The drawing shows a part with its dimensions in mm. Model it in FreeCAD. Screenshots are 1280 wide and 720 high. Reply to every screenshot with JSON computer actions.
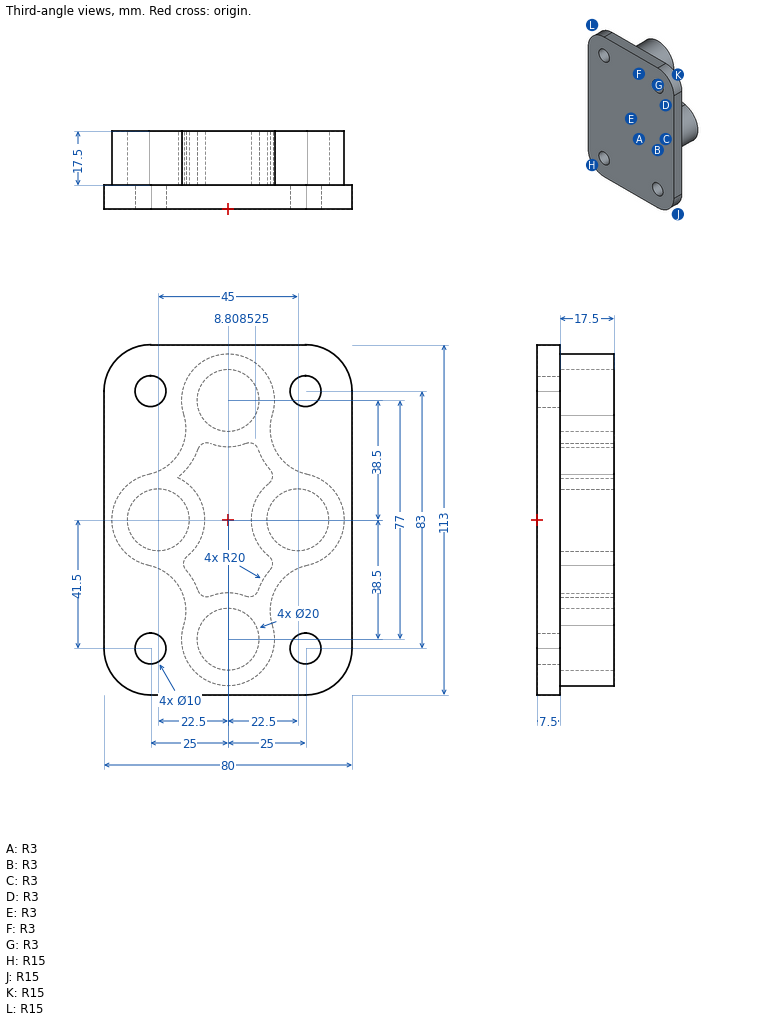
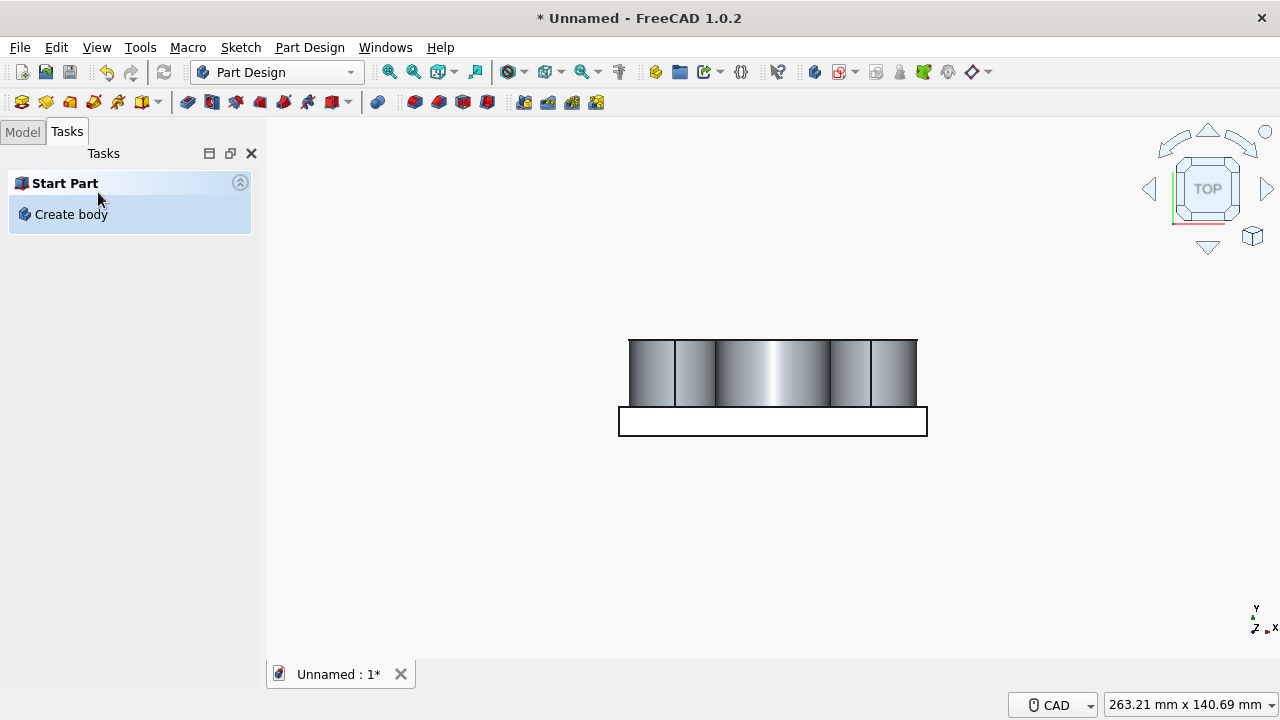
{"action": "left_click", "coordinate": [390, 72]}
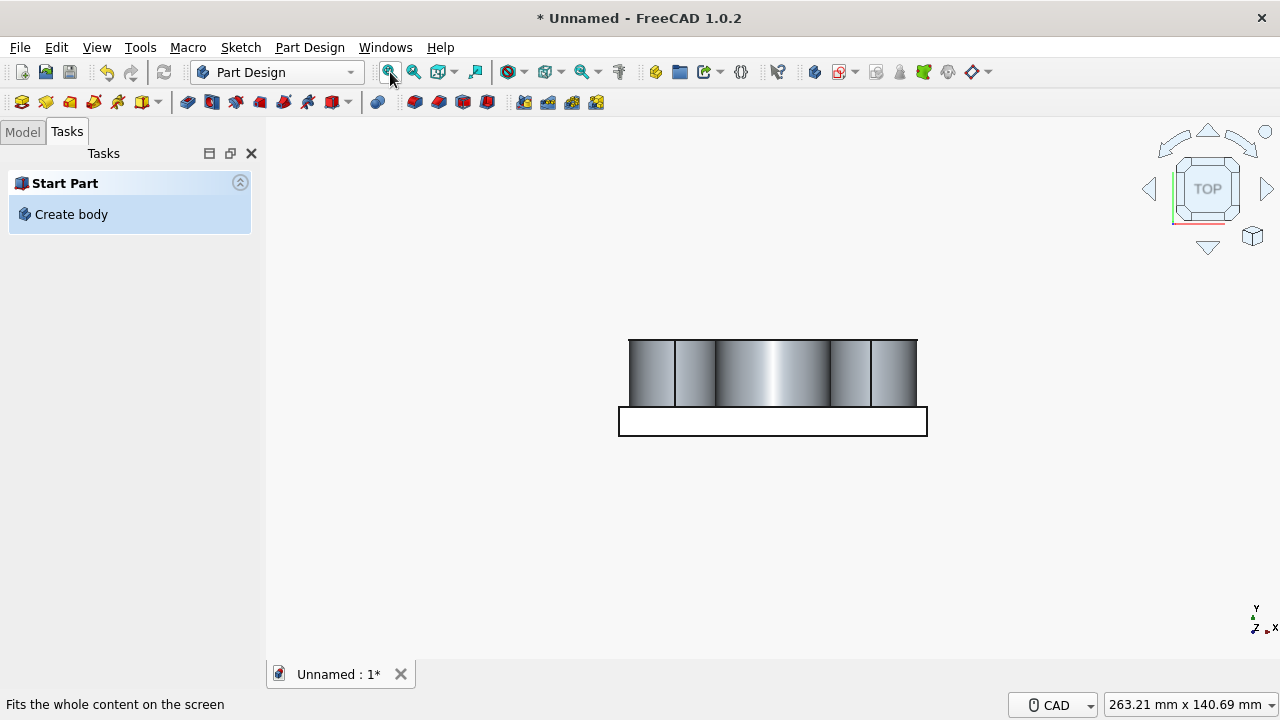
{"action": "key", "text": "0"}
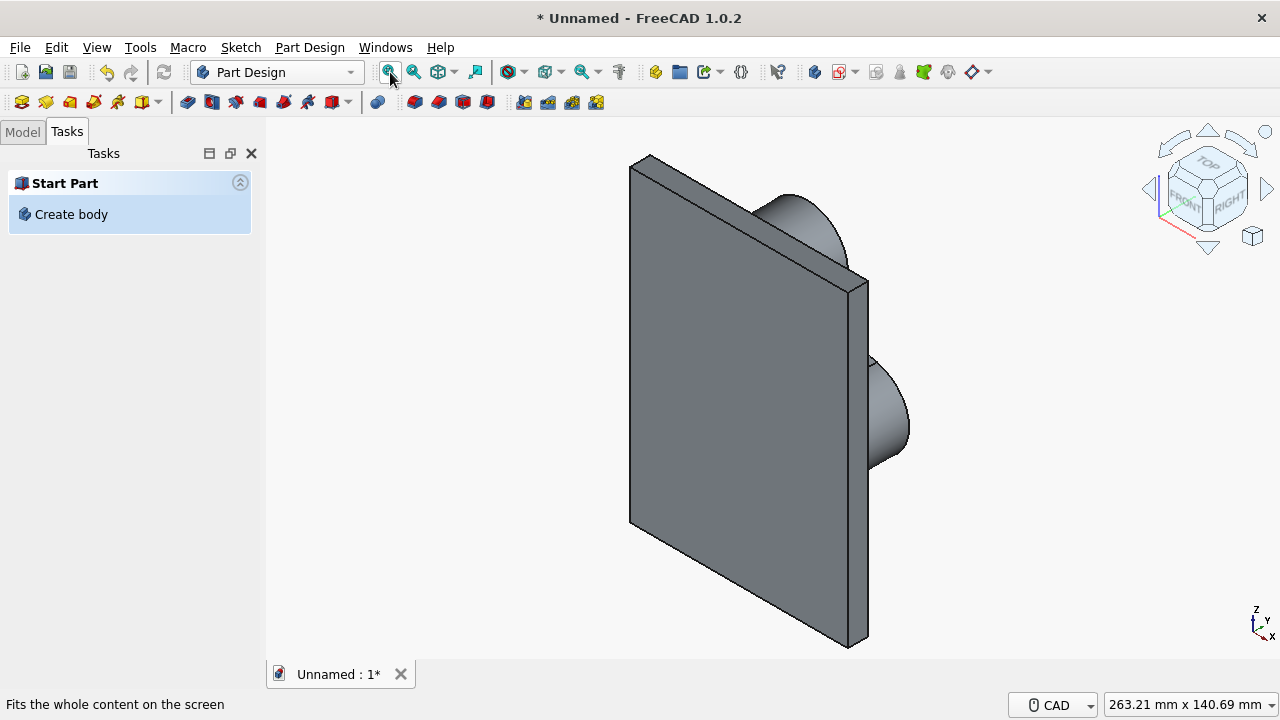
{"action": "key", "text": "1"}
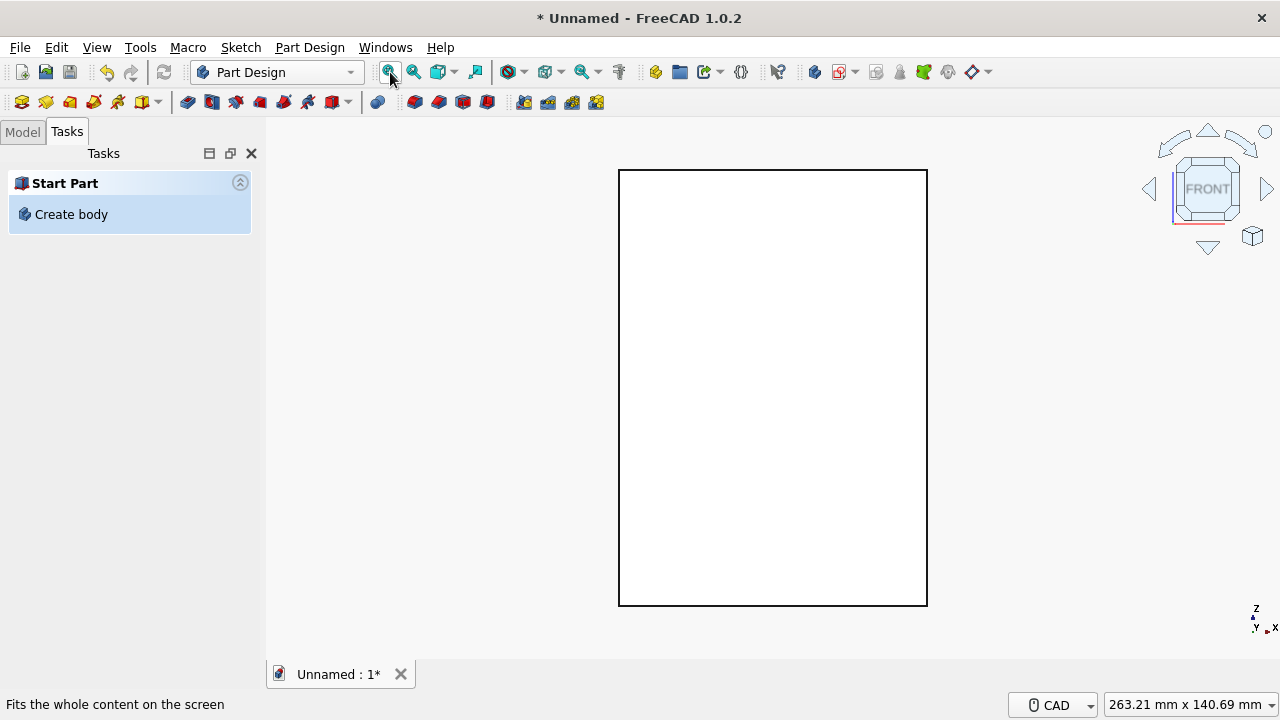
{"action": "key", "text": "3"}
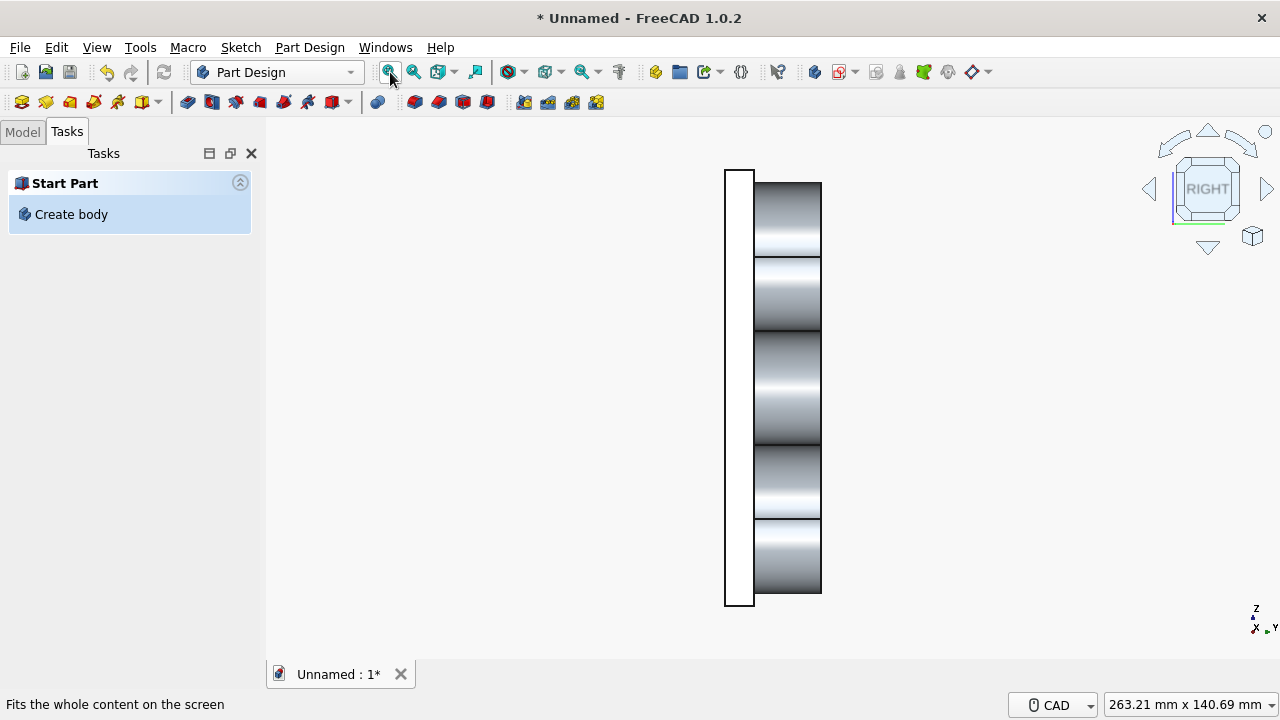
{"action": "key", "text": "5"}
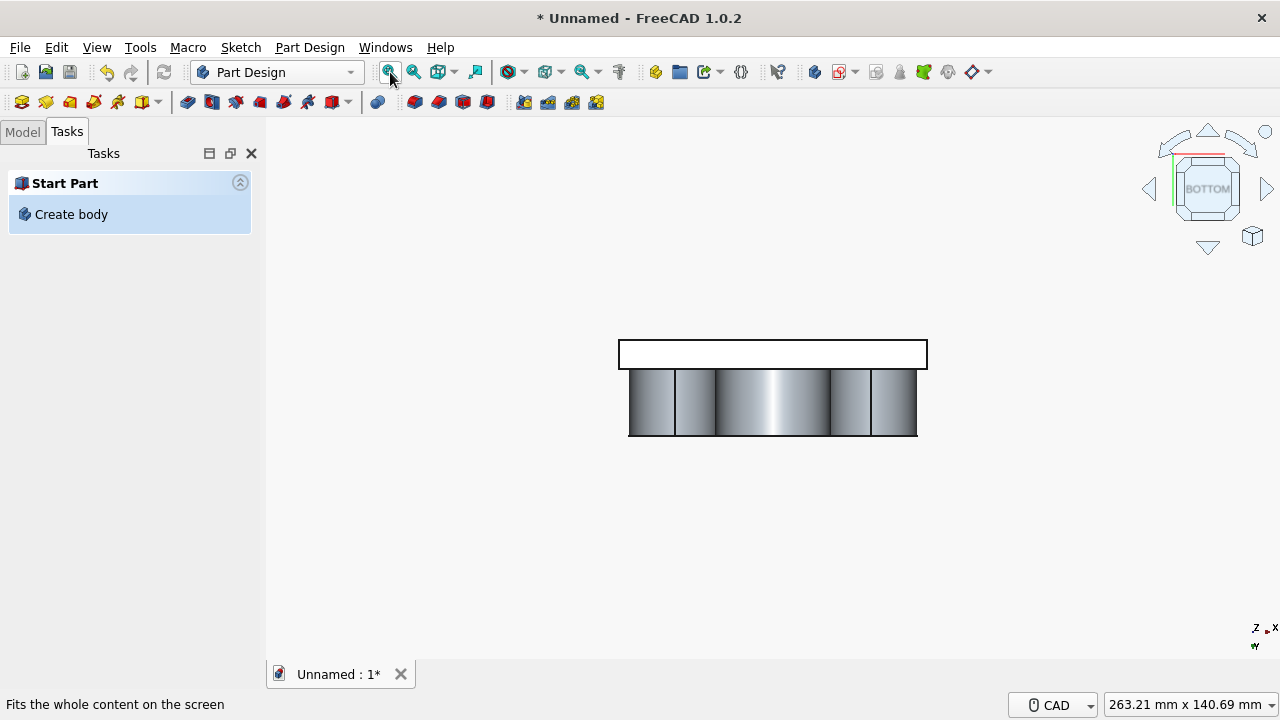
{"action": "left_click", "coordinate": [390, 72]}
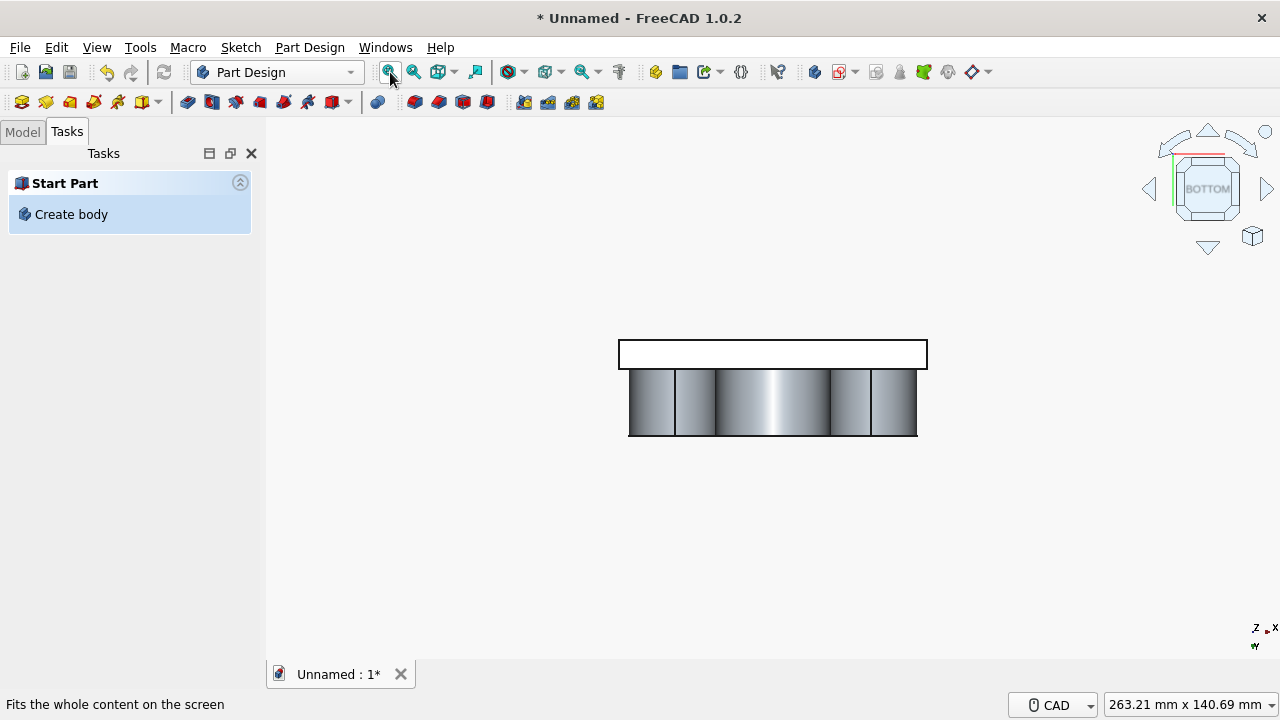
{"action": "key", "text": "4"}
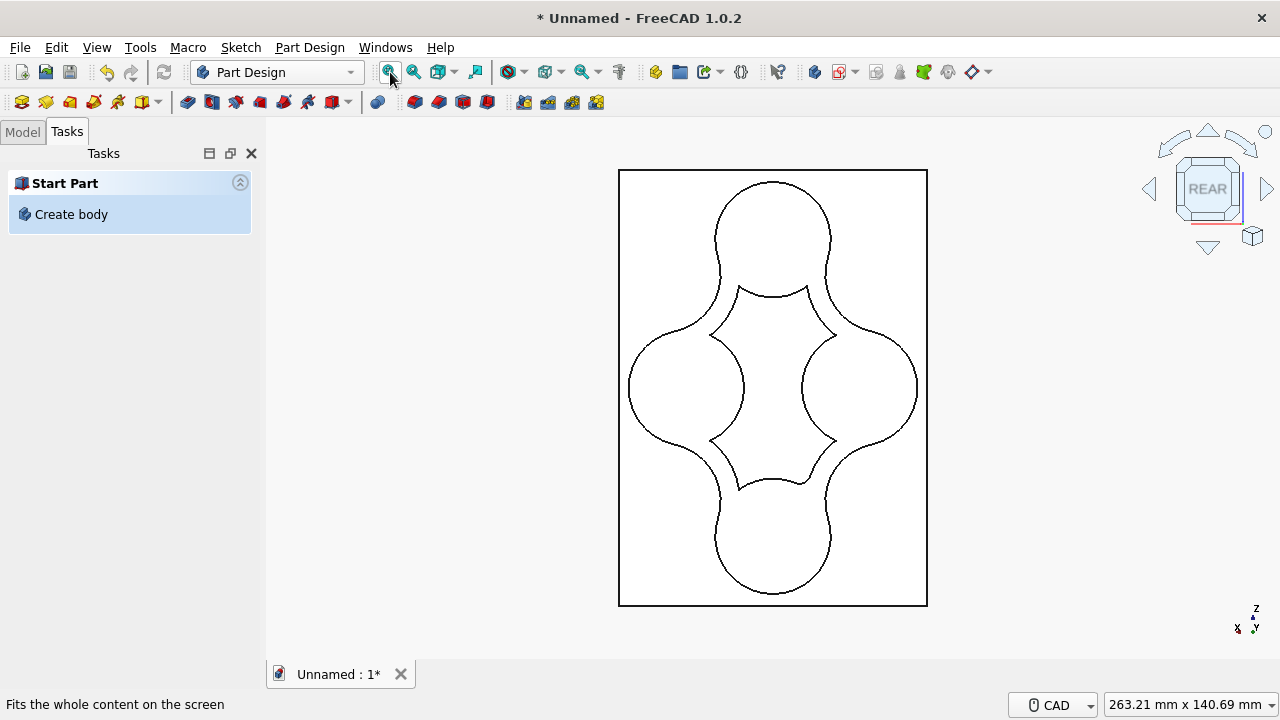
{"action": "key", "text": "6"}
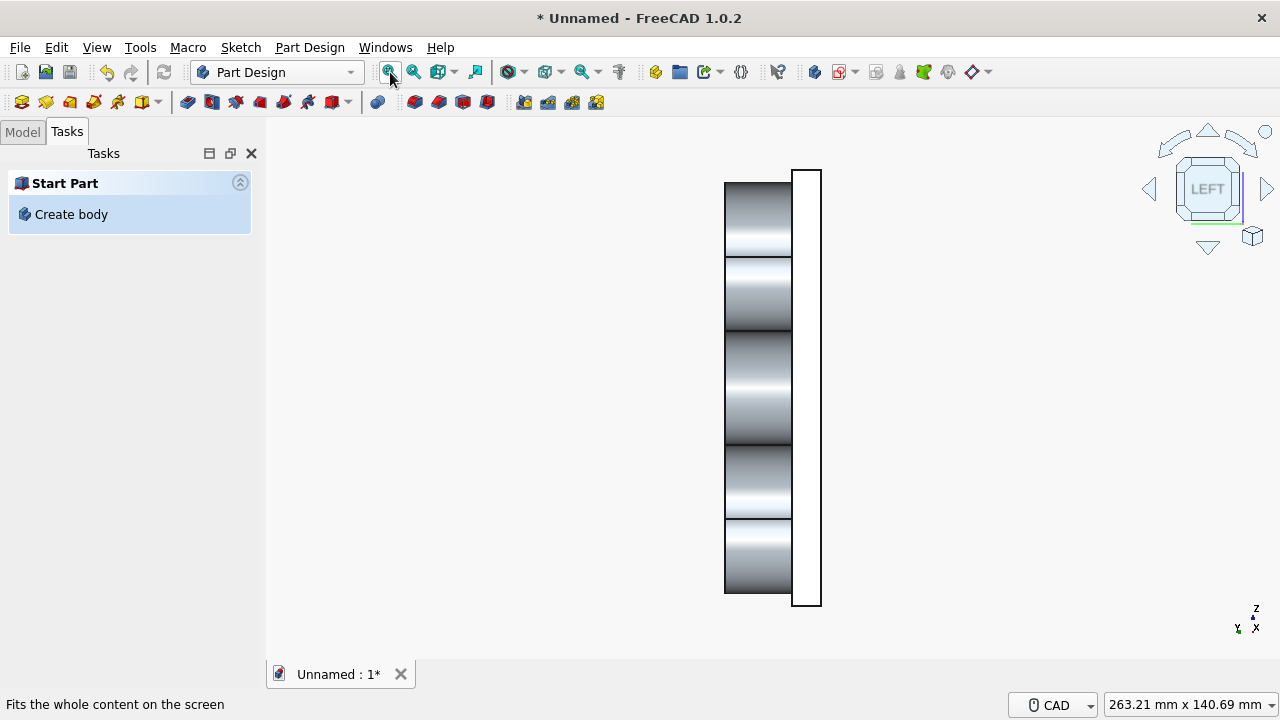
{"action": "key", "text": "v 3"}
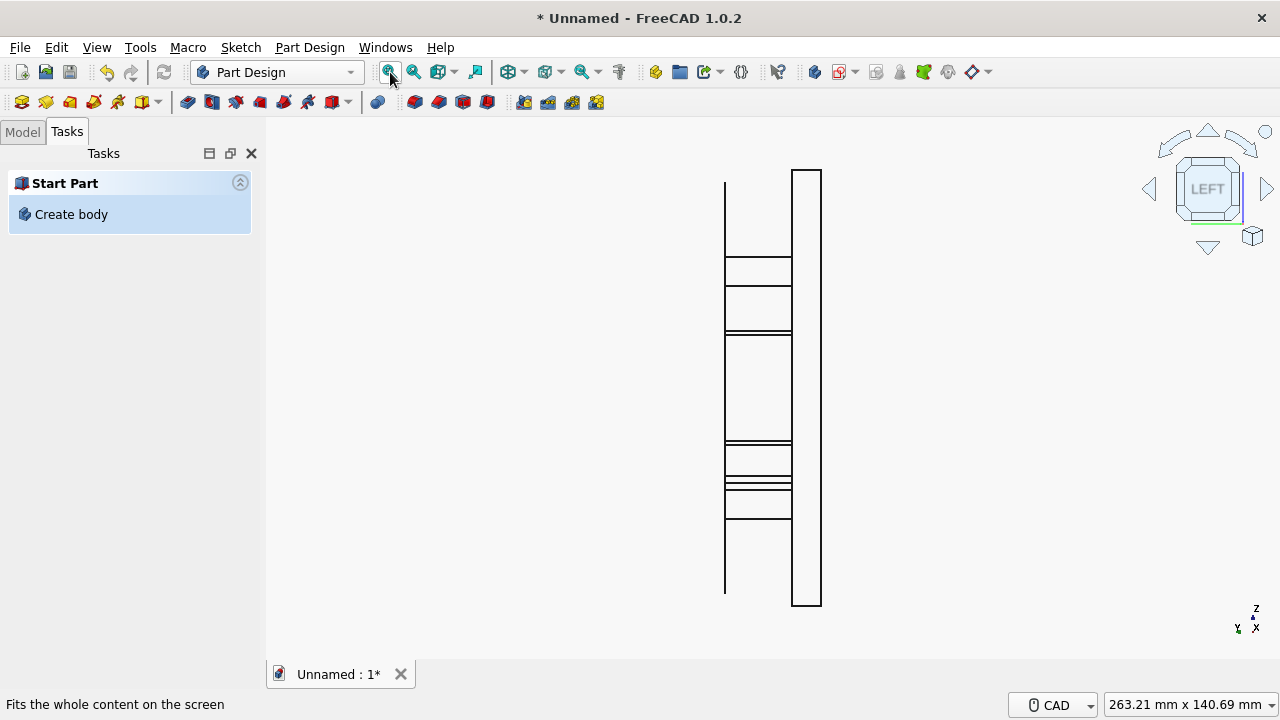
{"action": "key", "text": "0"}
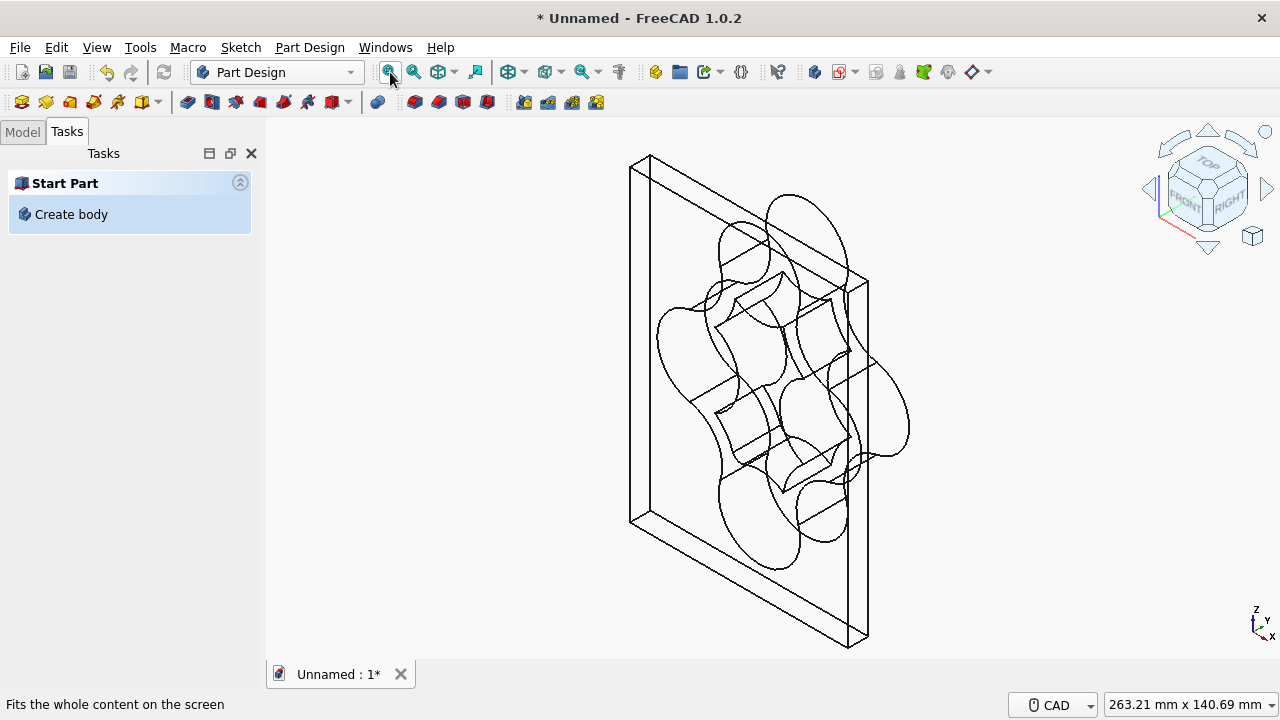
{"action": "left_click", "coordinate": [817, 472]}